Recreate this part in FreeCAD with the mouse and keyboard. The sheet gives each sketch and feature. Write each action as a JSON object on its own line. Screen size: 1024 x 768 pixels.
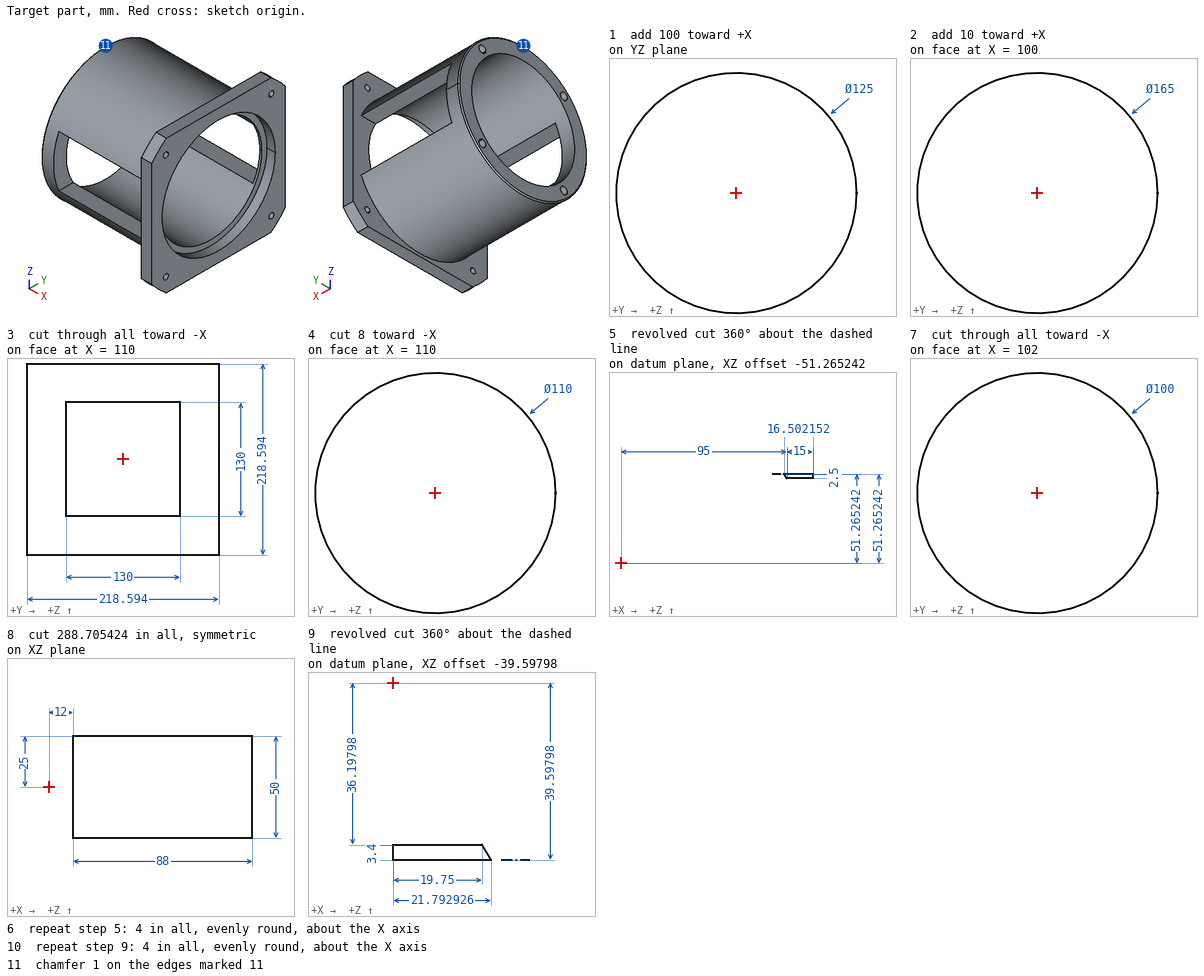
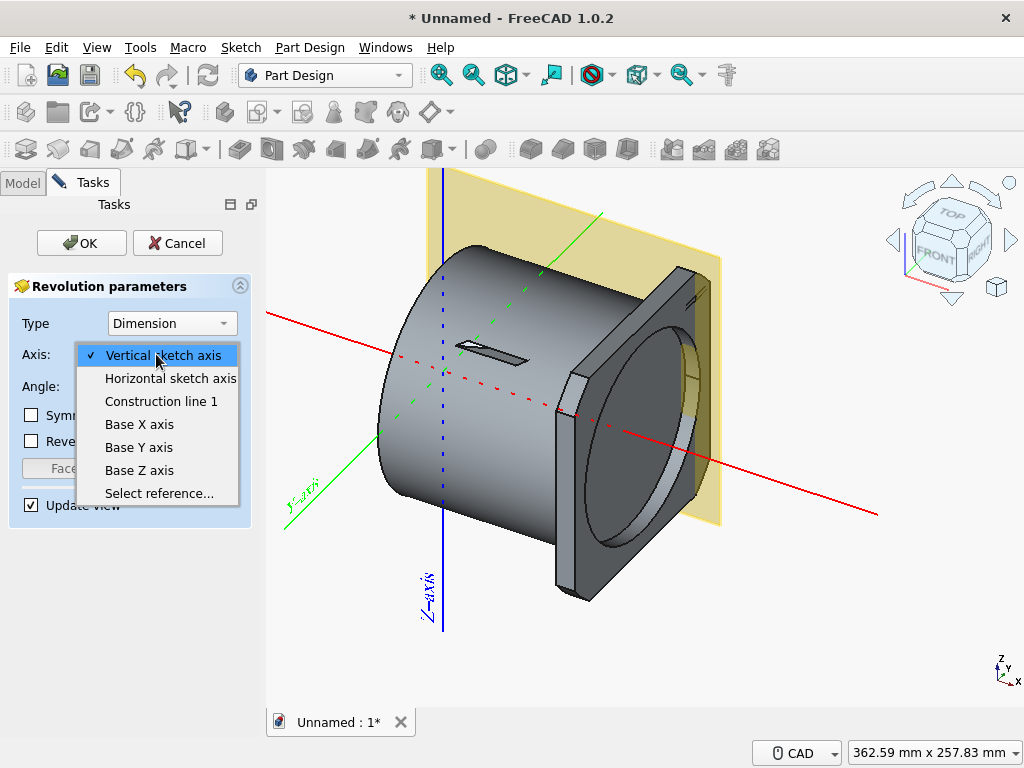
{"action": "left_click", "coordinate": [156, 402]}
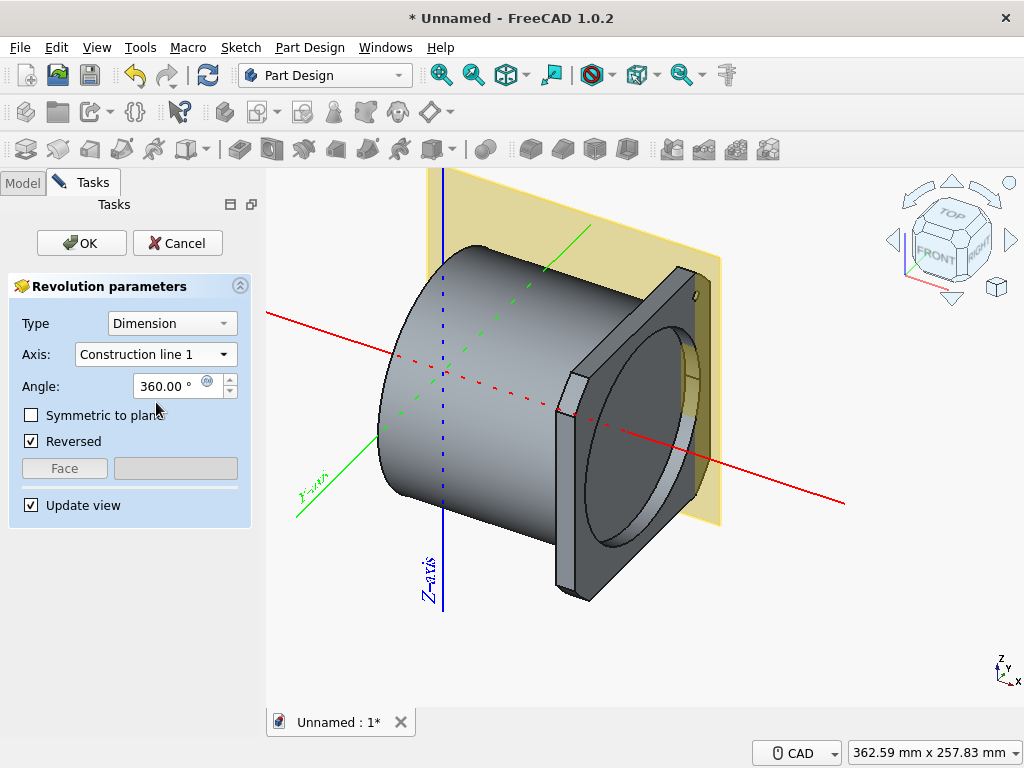
{"action": "left_click", "coordinate": [82, 243]}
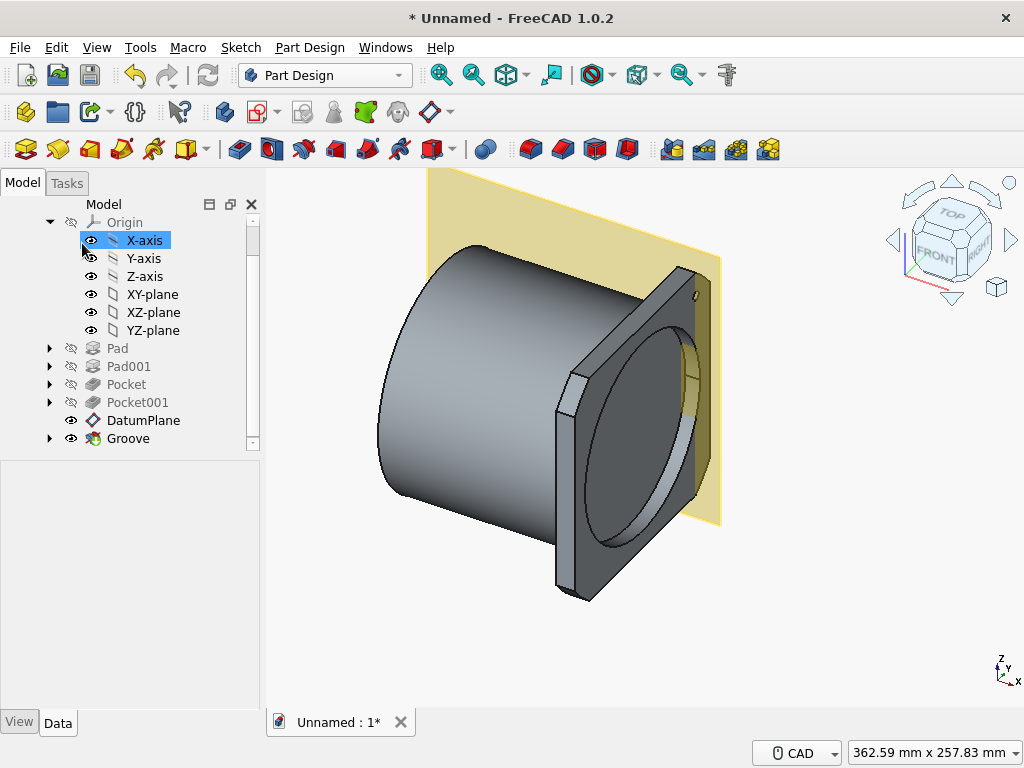
{"action": "left_click", "coordinate": [116, 420]}
{"action": "key", "text": "space"}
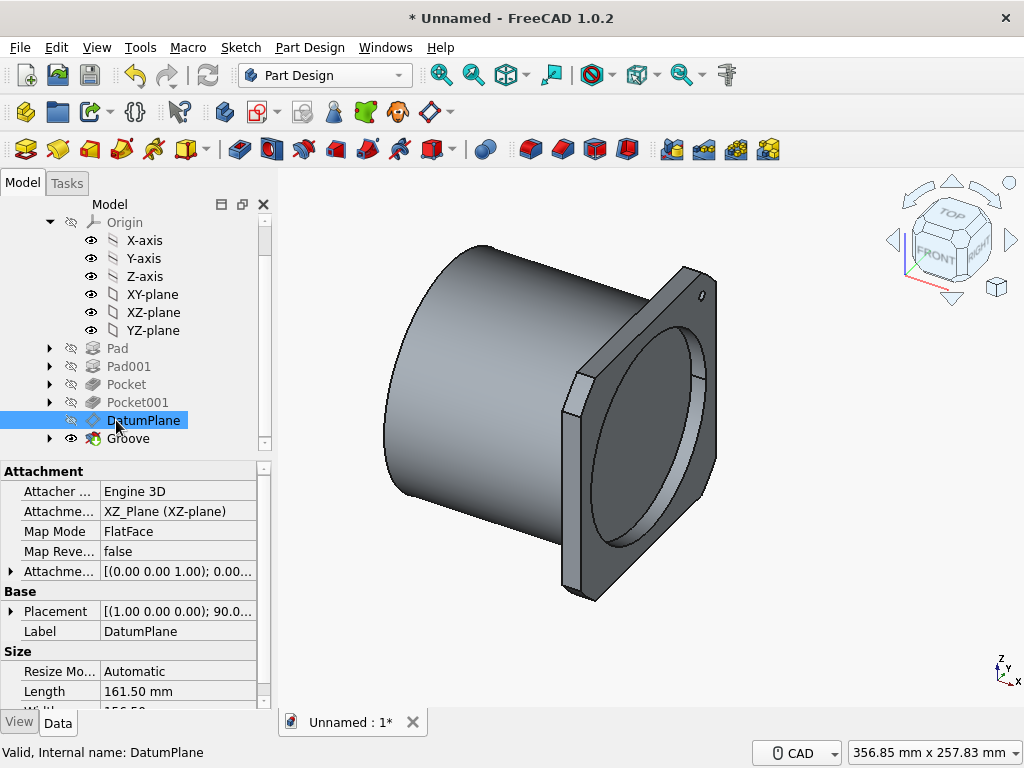
{"action": "left_click", "coordinate": [116, 438]}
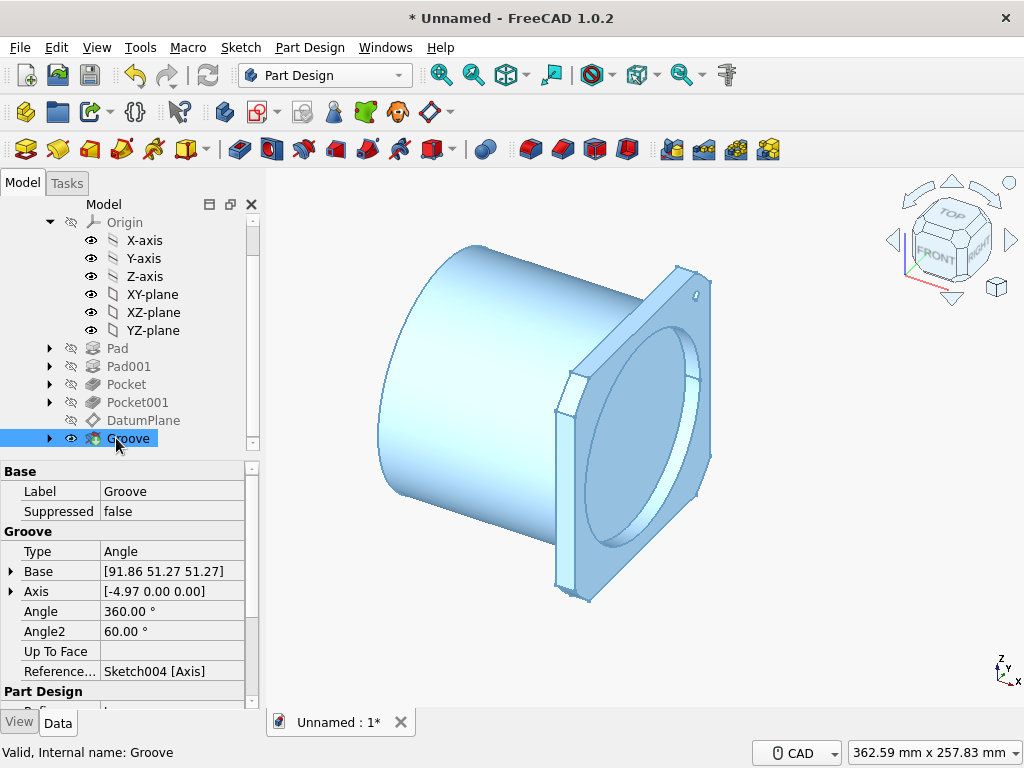
{"action": "left_click", "coordinate": [736, 150]}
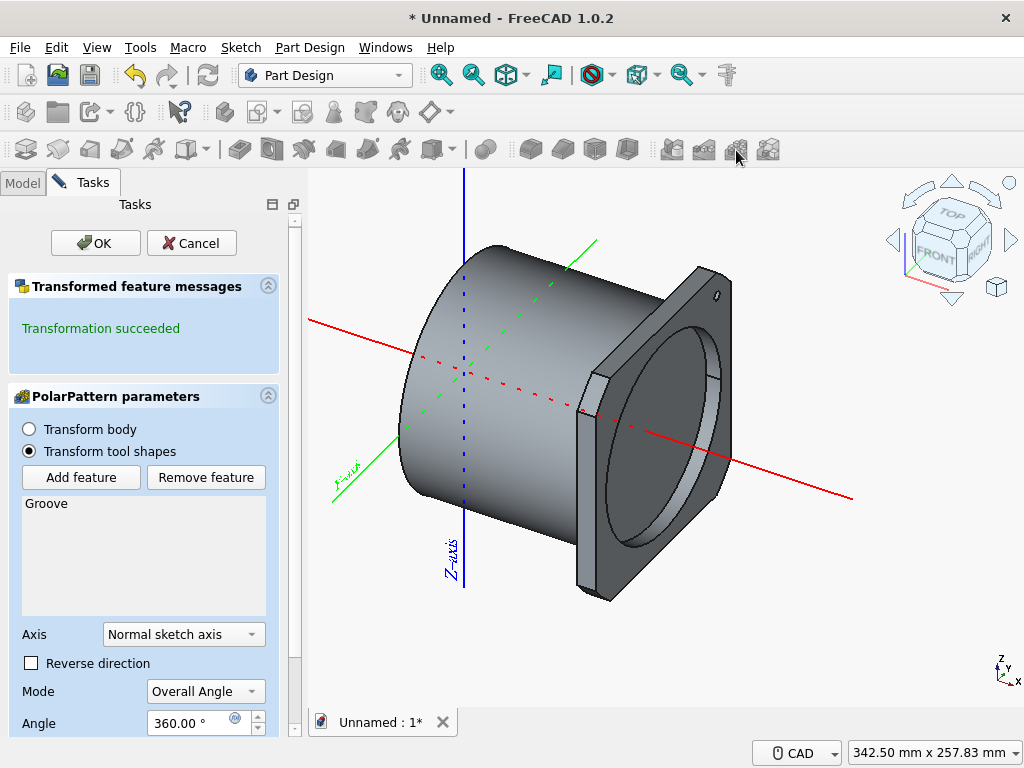
{"action": "left_click", "coordinate": [184, 634]}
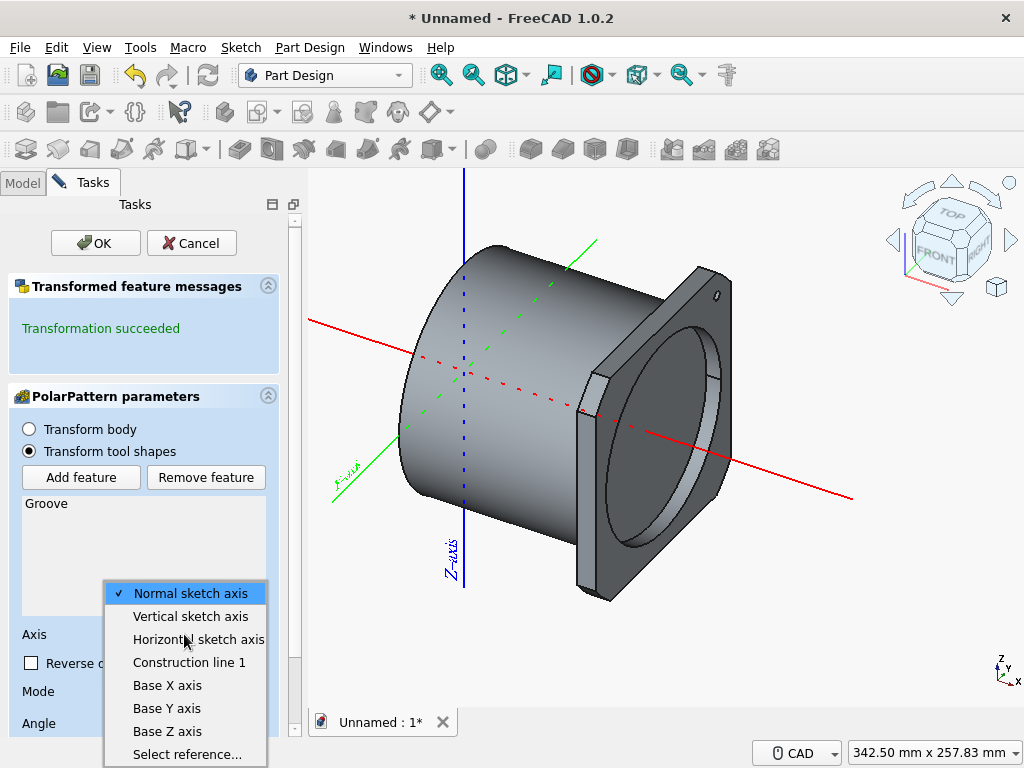
{"action": "left_click", "coordinate": [184, 686]}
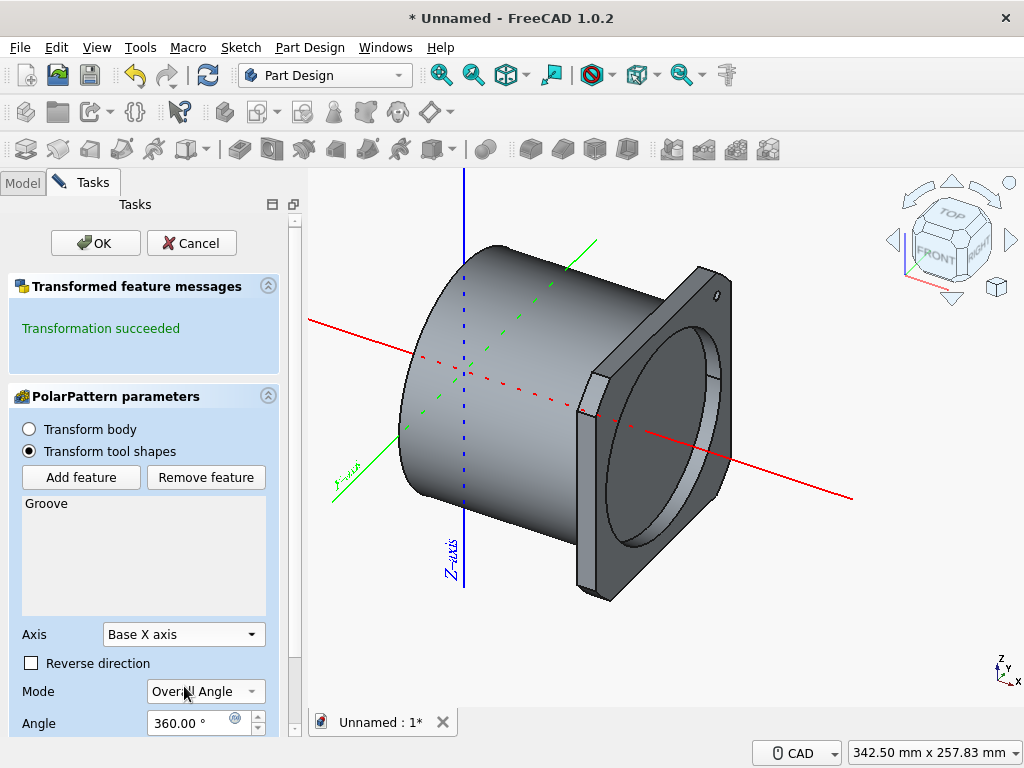
{"action": "scroll", "coordinate": [295, 475], "scroll_direction": "down", "scroll_amount": 2}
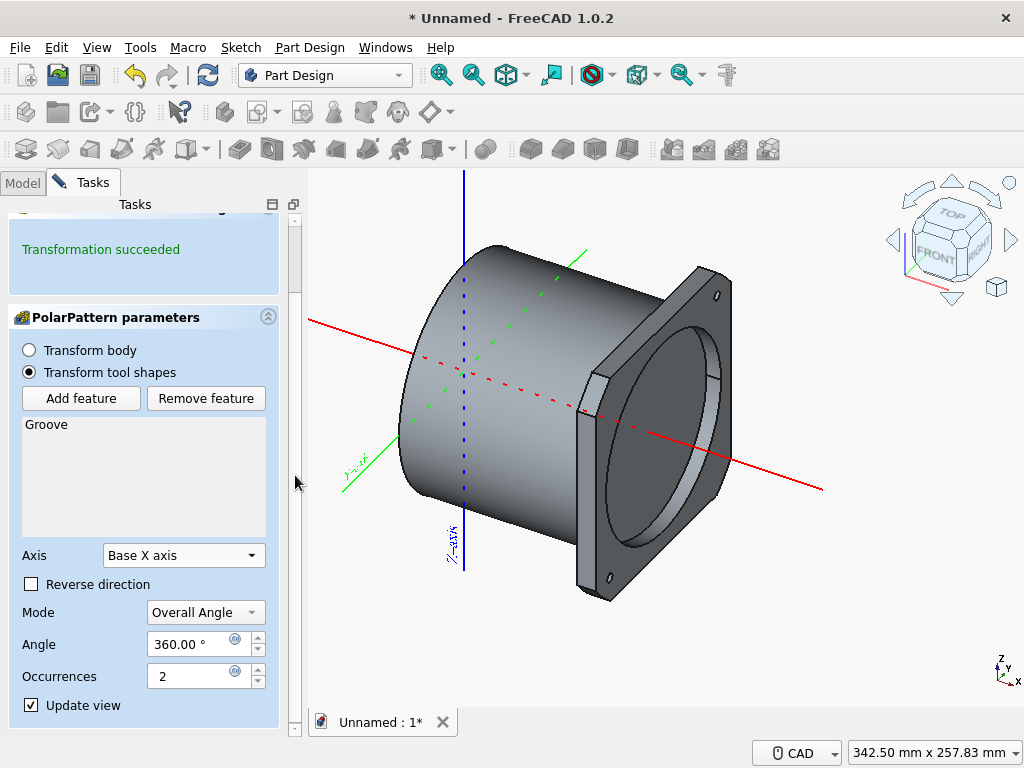
{"action": "triple_click", "coordinate": [198, 676]}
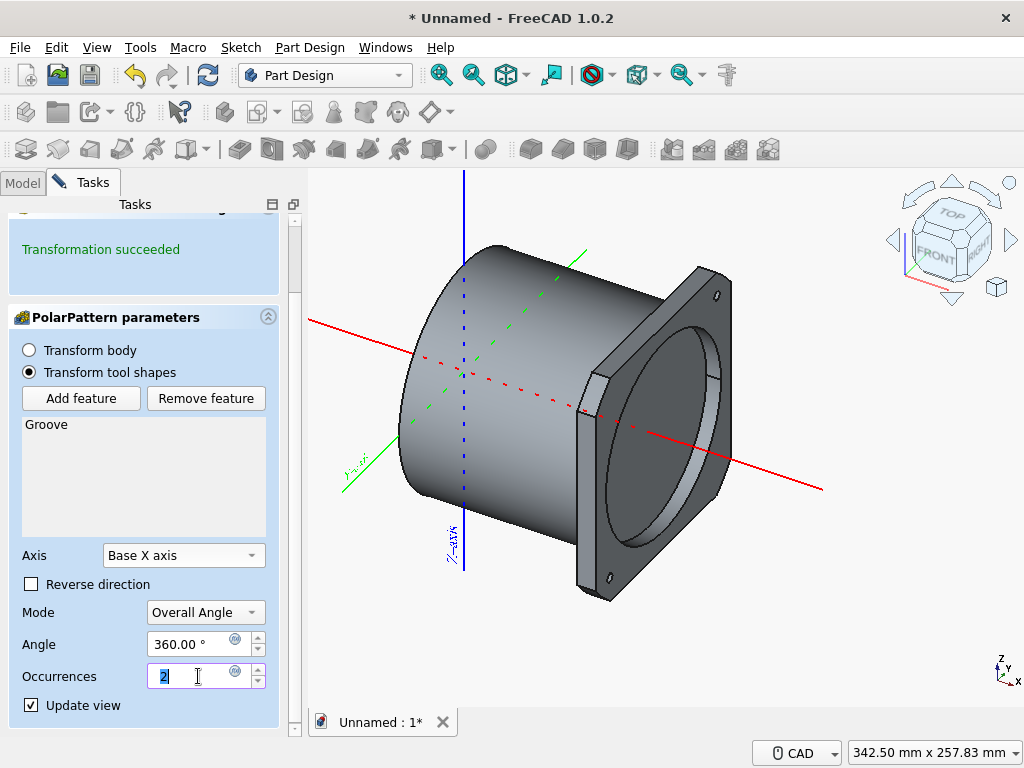
{"action": "type", "text": "4"}
{"action": "key", "text": "Tab"}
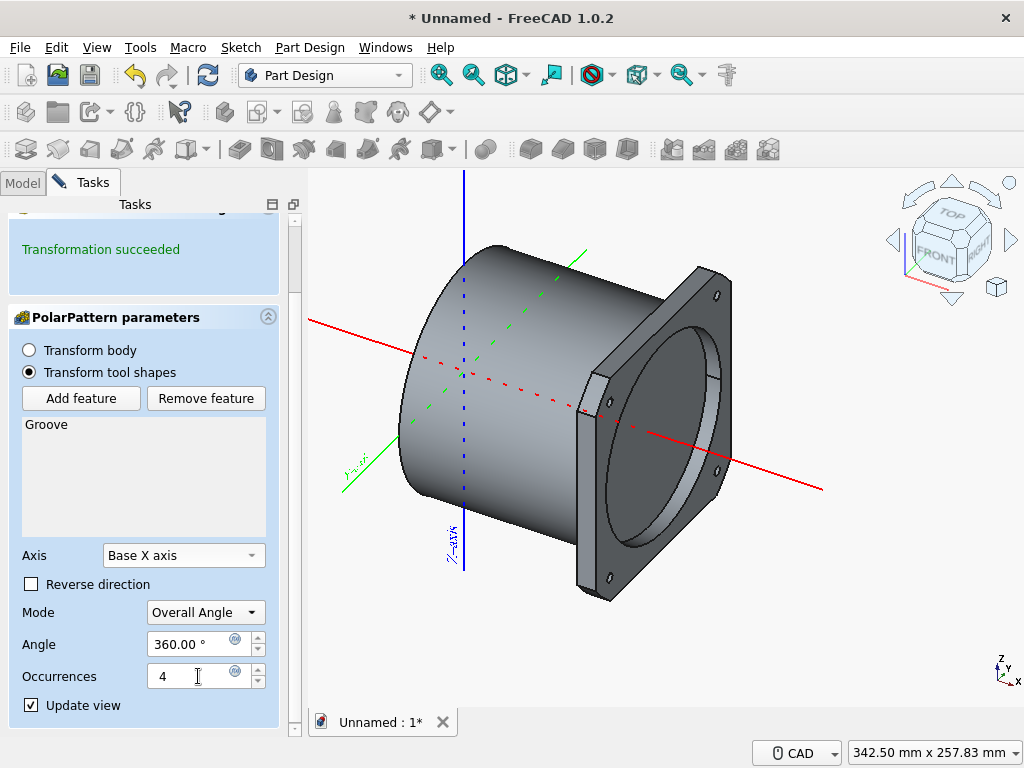
{"action": "scroll", "coordinate": [295, 475], "scroll_direction": "up", "scroll_amount": 3}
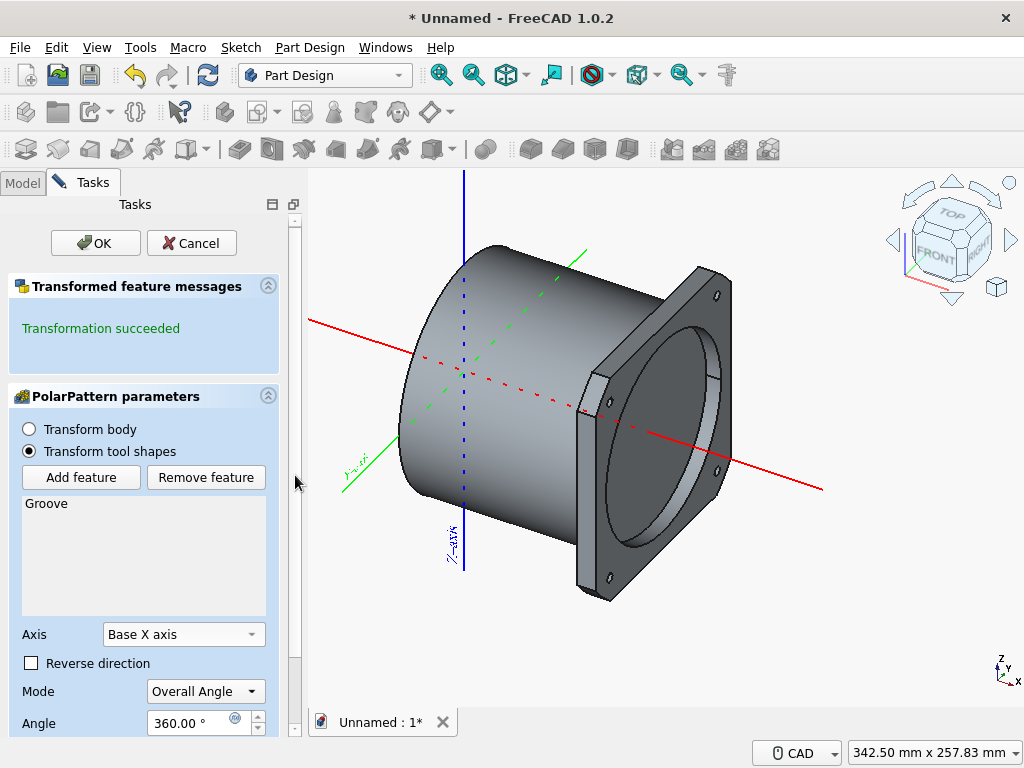
{"action": "left_click", "coordinate": [96, 243]}